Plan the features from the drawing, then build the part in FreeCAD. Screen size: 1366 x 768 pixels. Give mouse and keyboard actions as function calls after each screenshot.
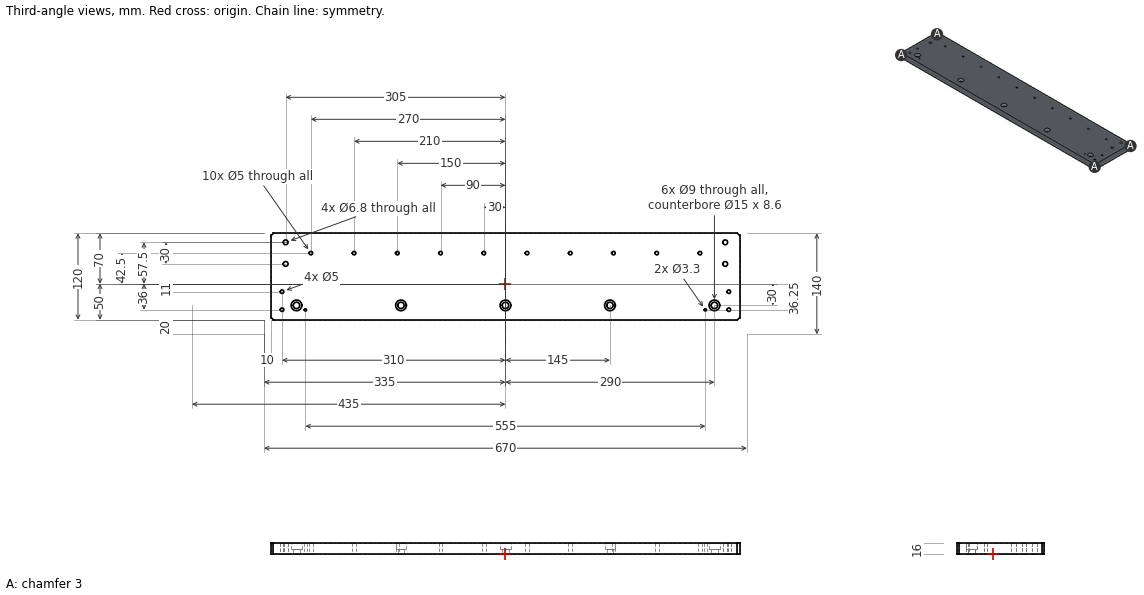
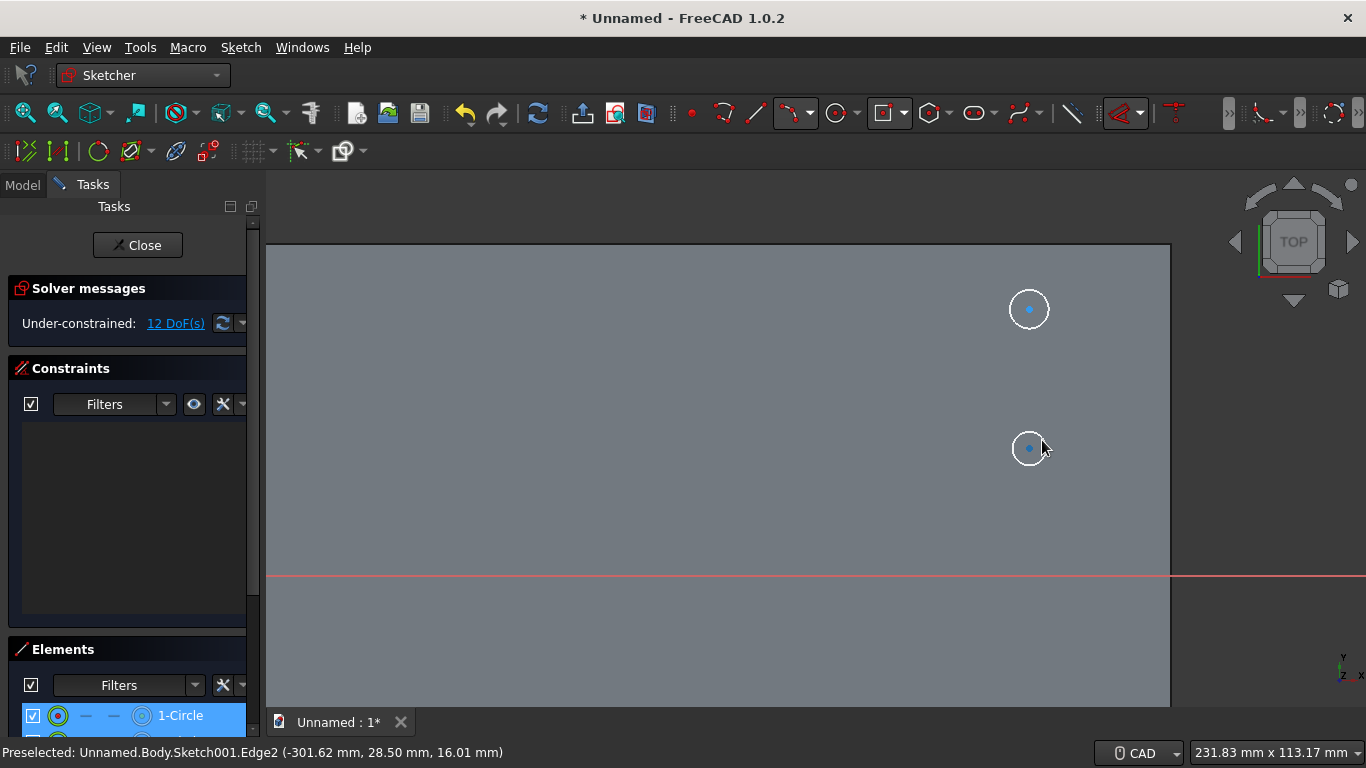
click(1041, 437)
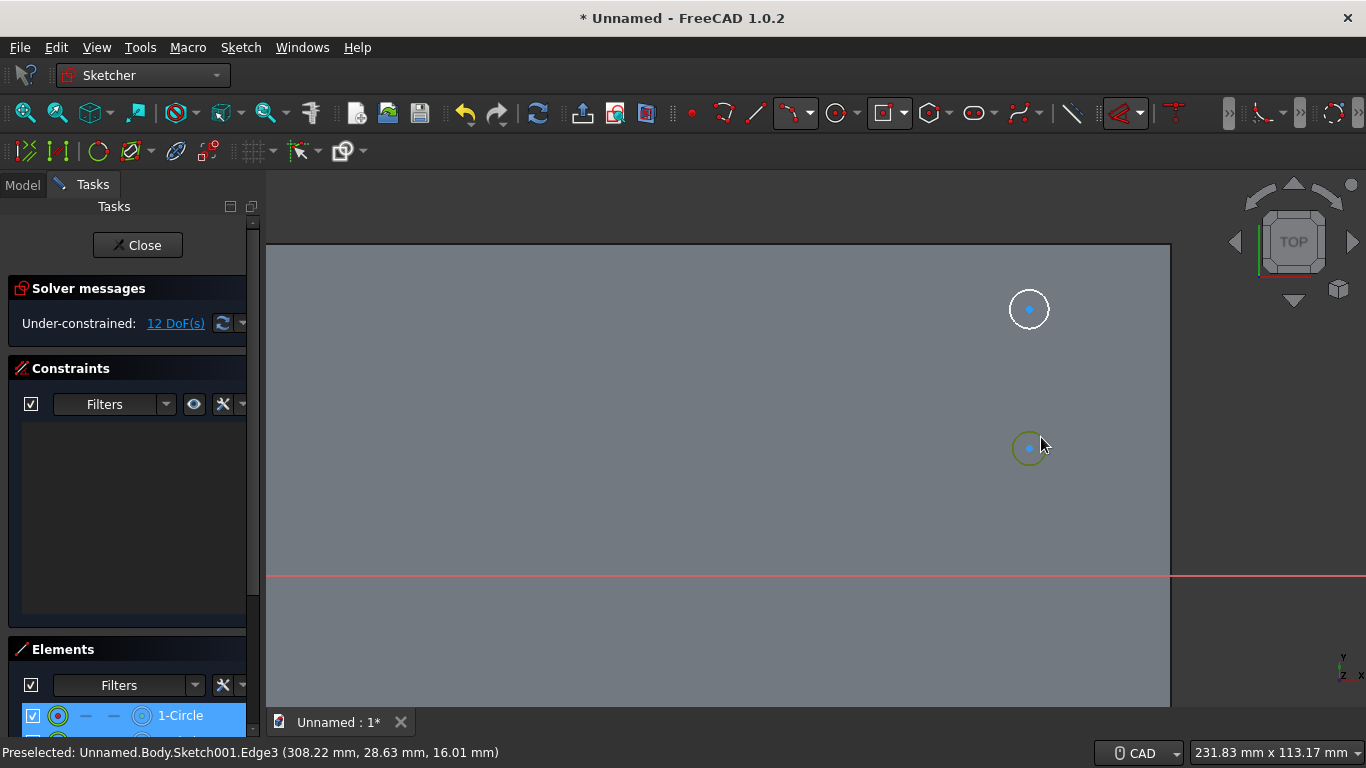
click(1043, 296)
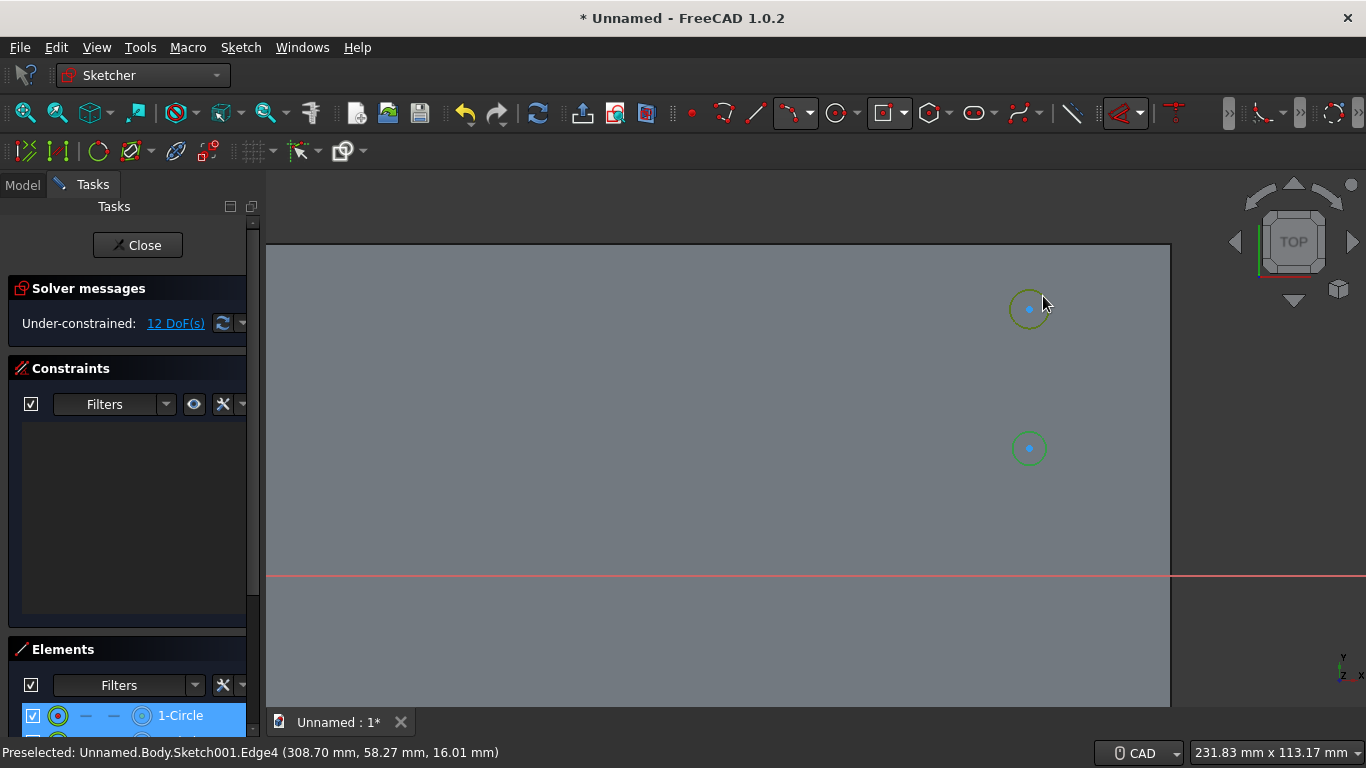
key(e)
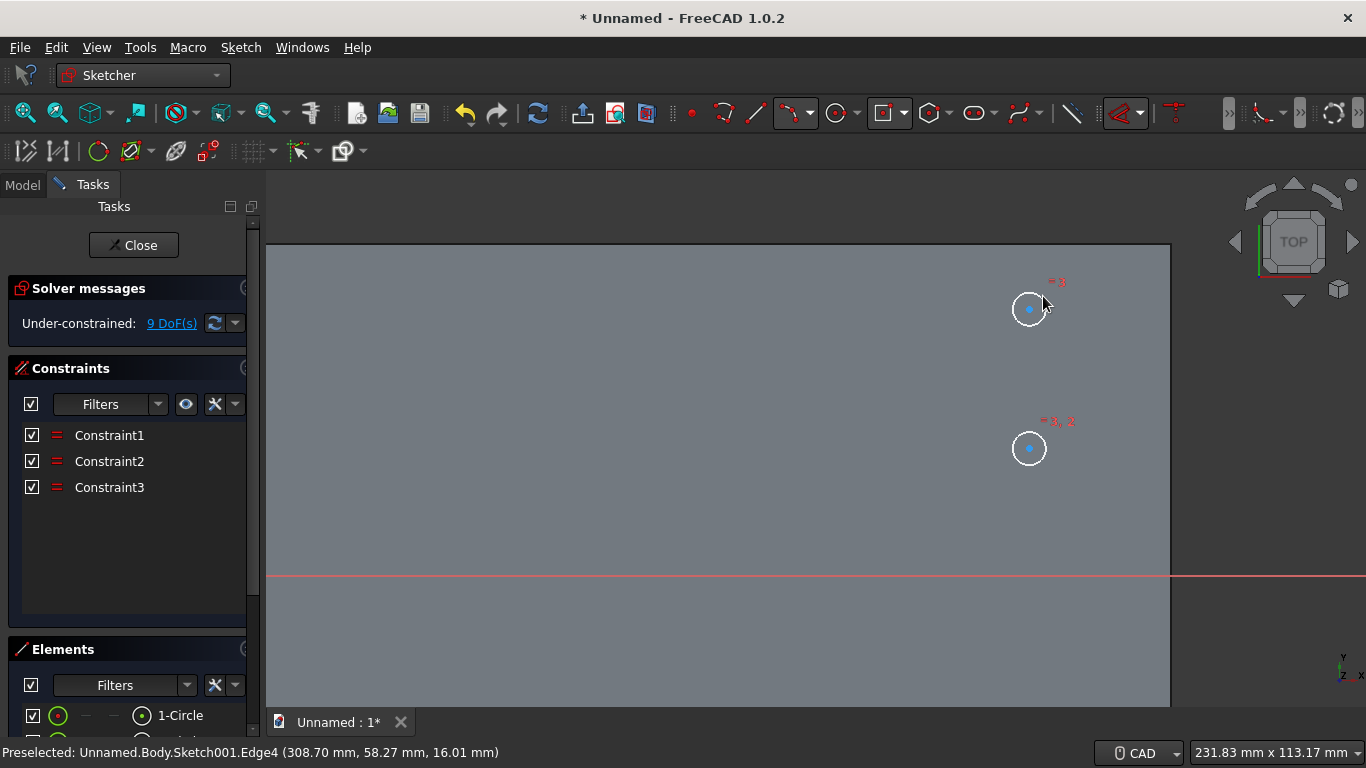
scroll(1042, 440, down, 8)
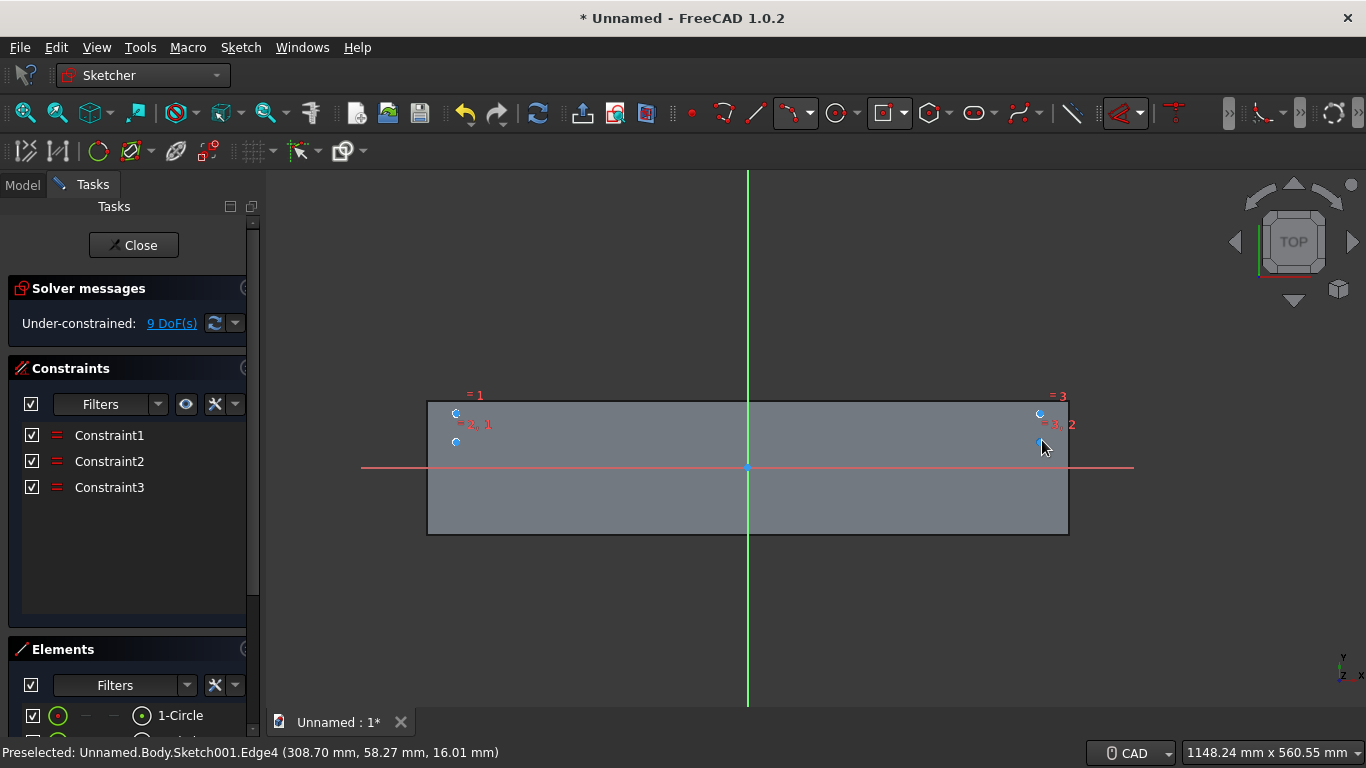
click(456, 442)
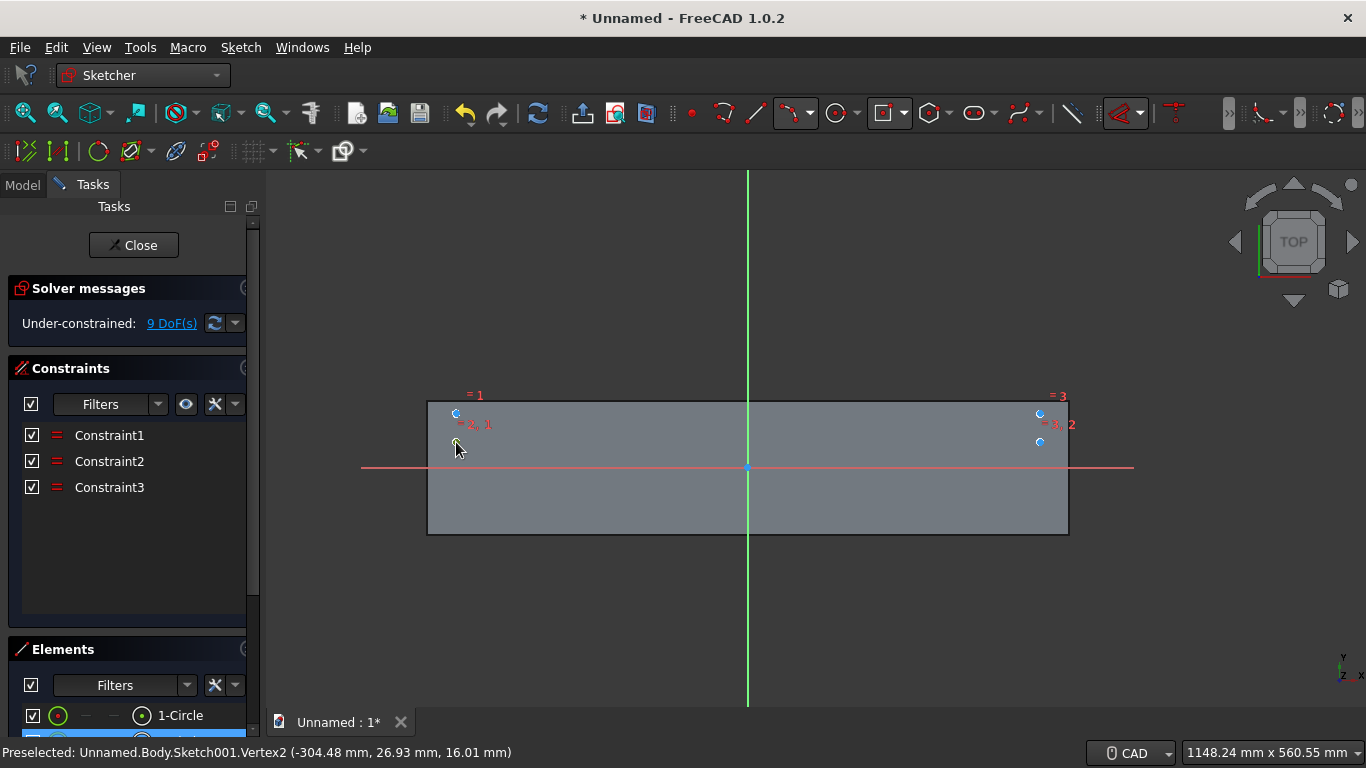
click(1040, 442)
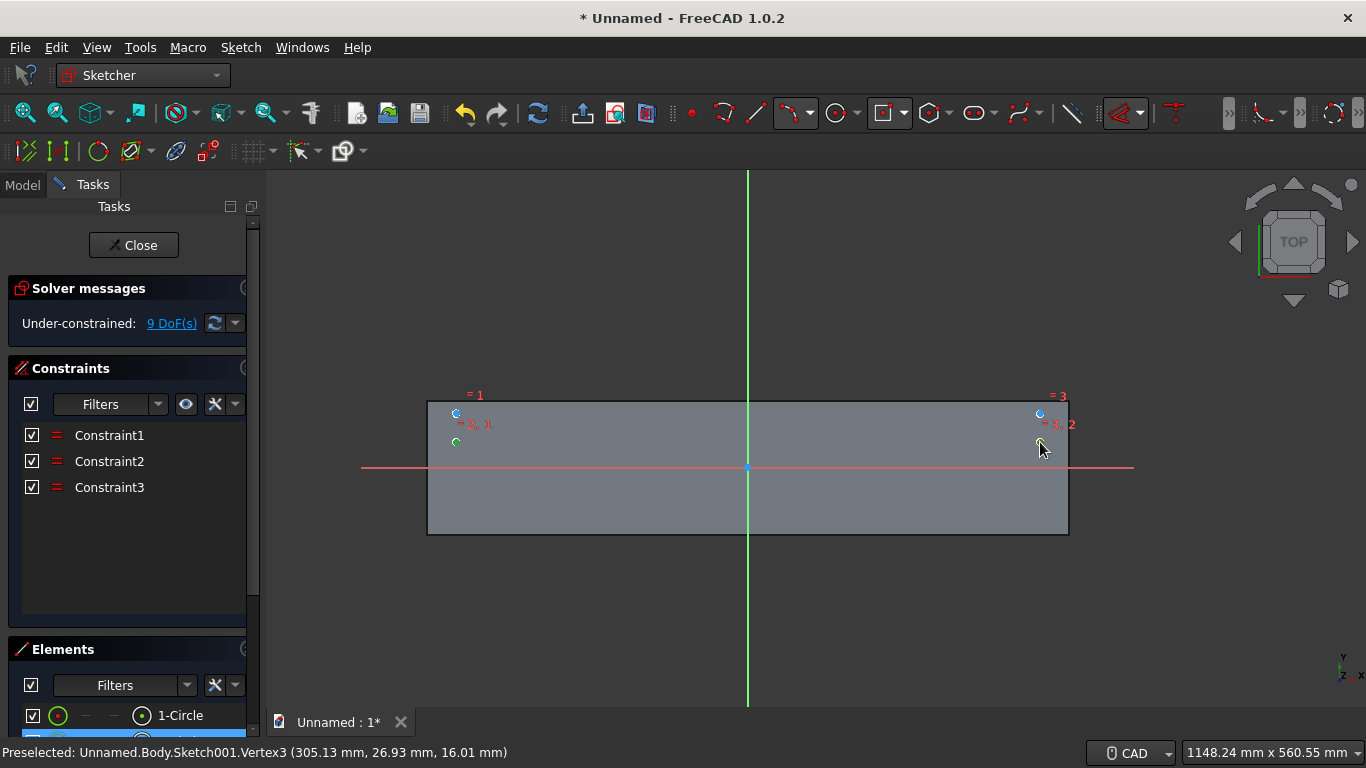
click(748, 645)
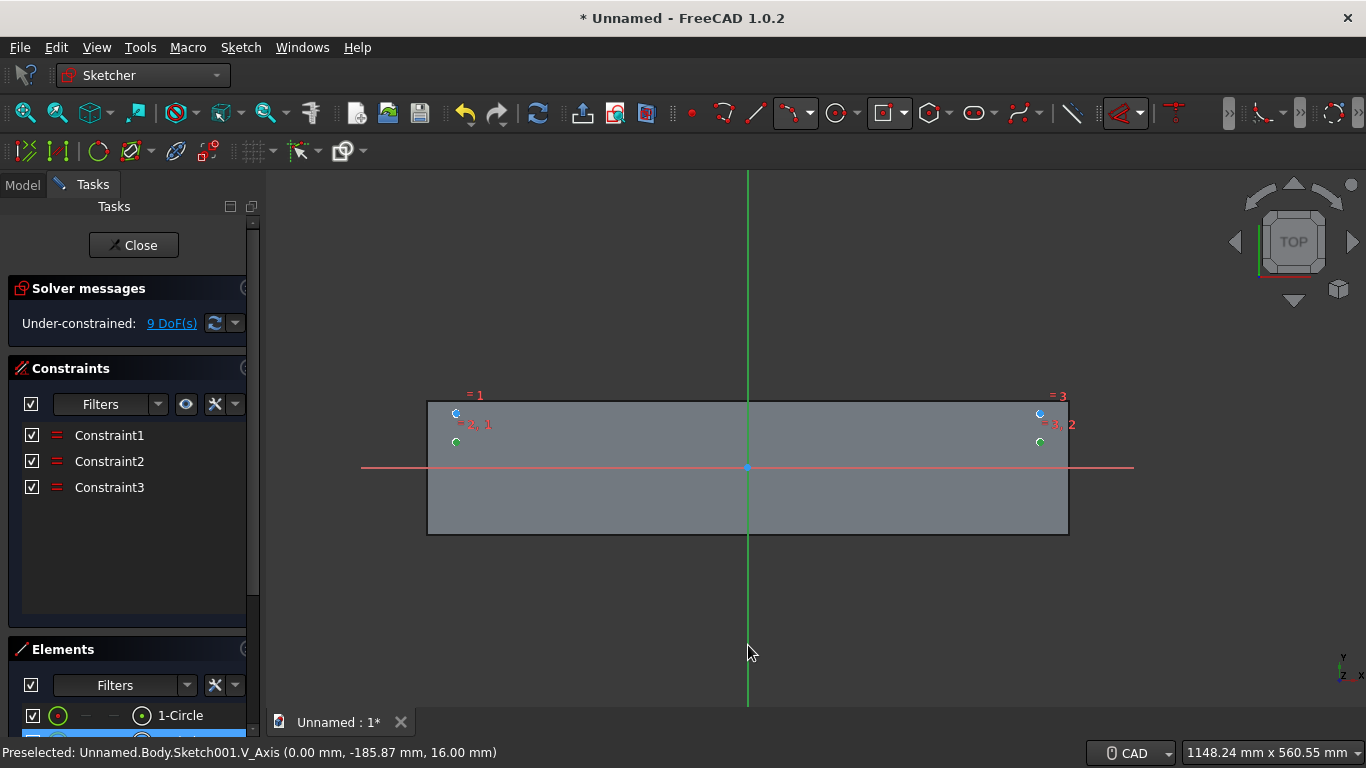
key(s)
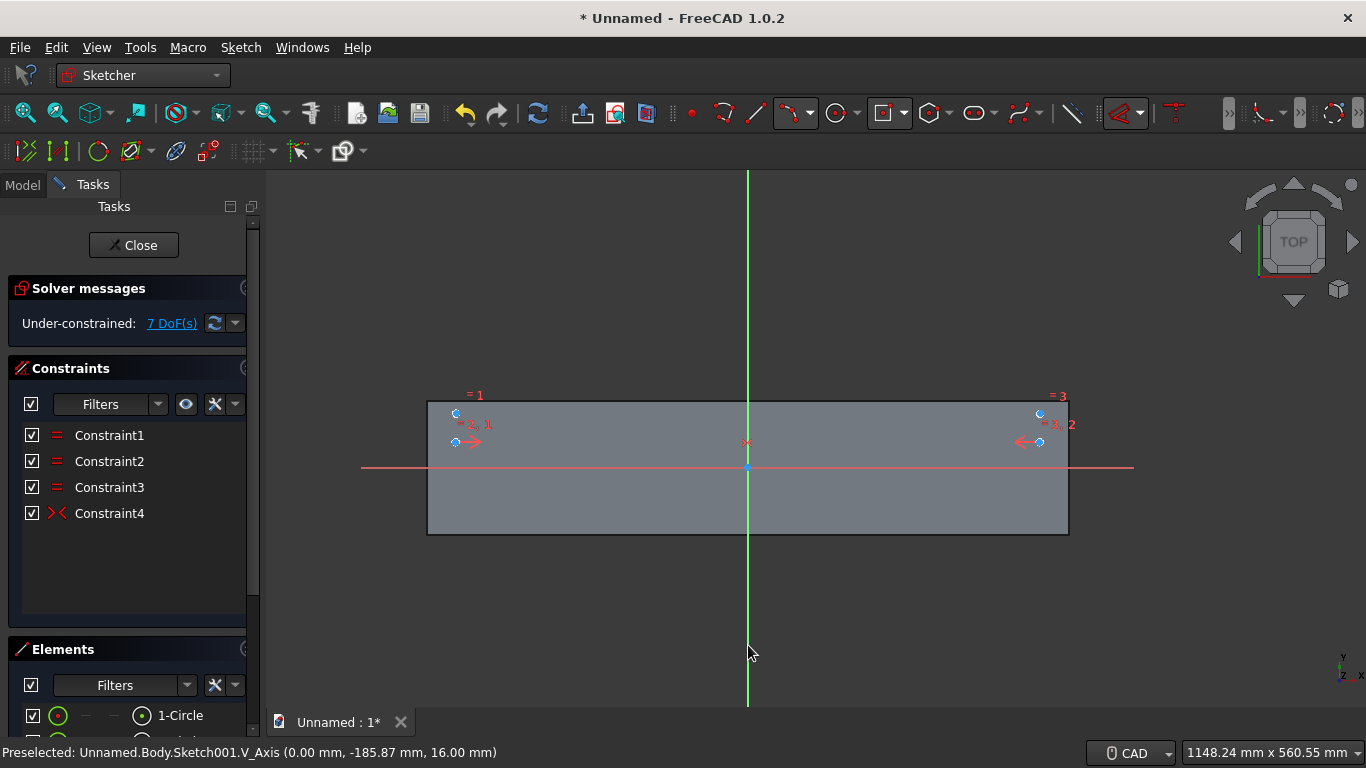
click(456, 414)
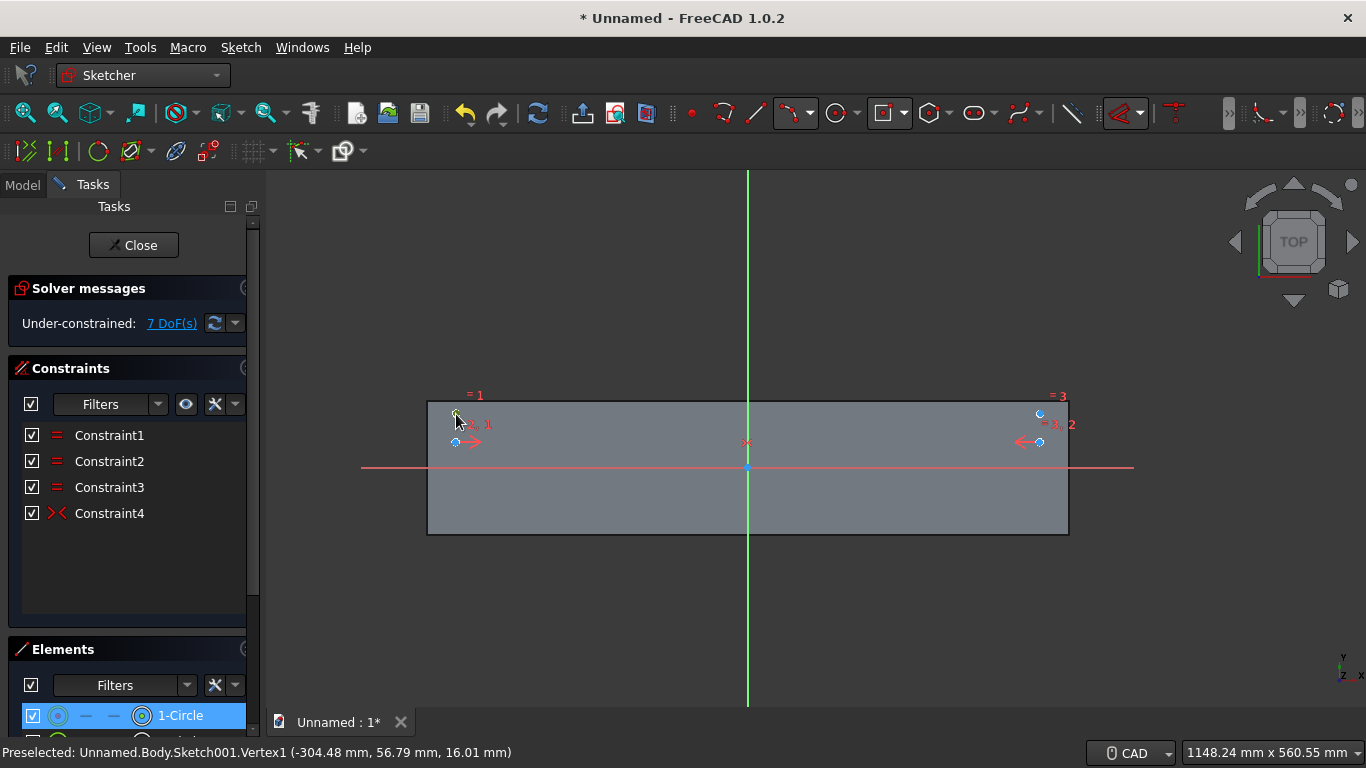
click(1040, 414)